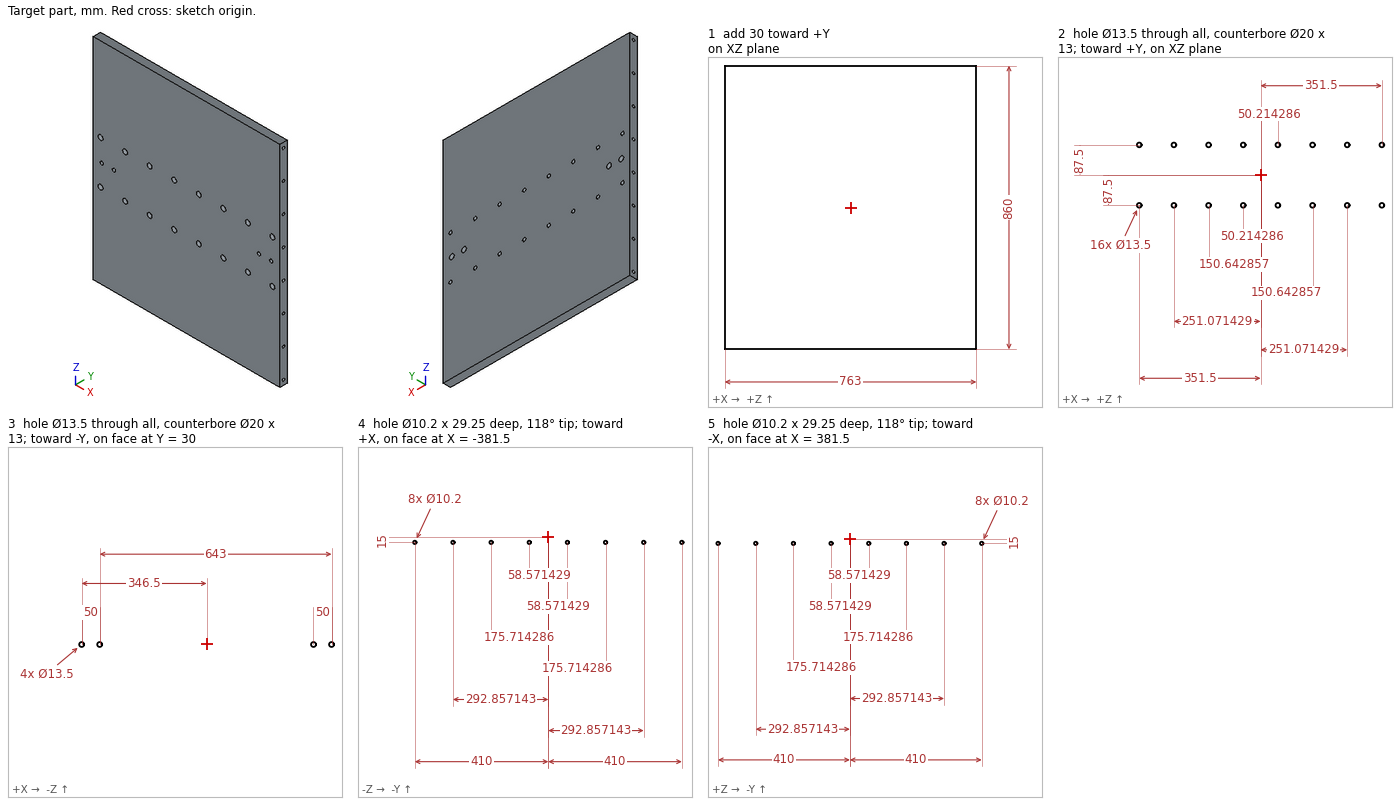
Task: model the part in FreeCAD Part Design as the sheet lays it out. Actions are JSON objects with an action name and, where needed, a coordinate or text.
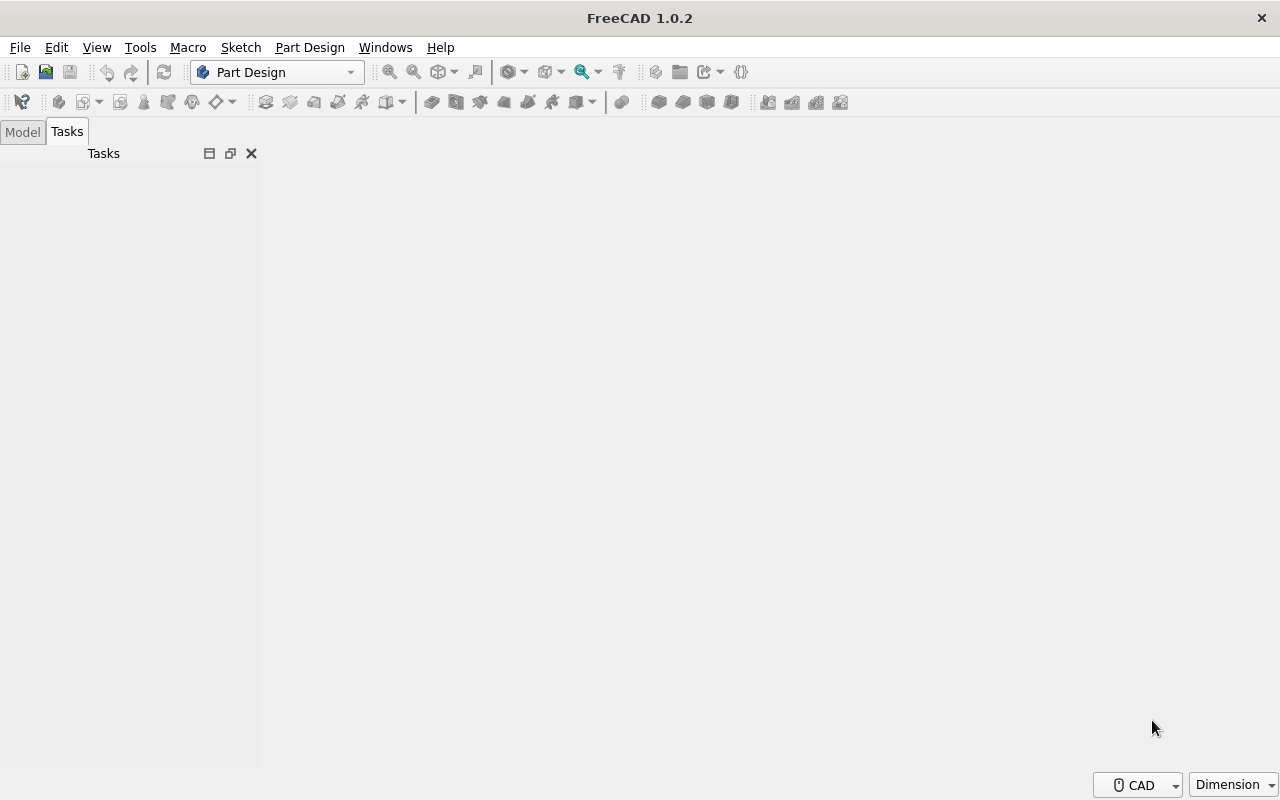
{"action": "left_click", "coordinate": [22, 72]}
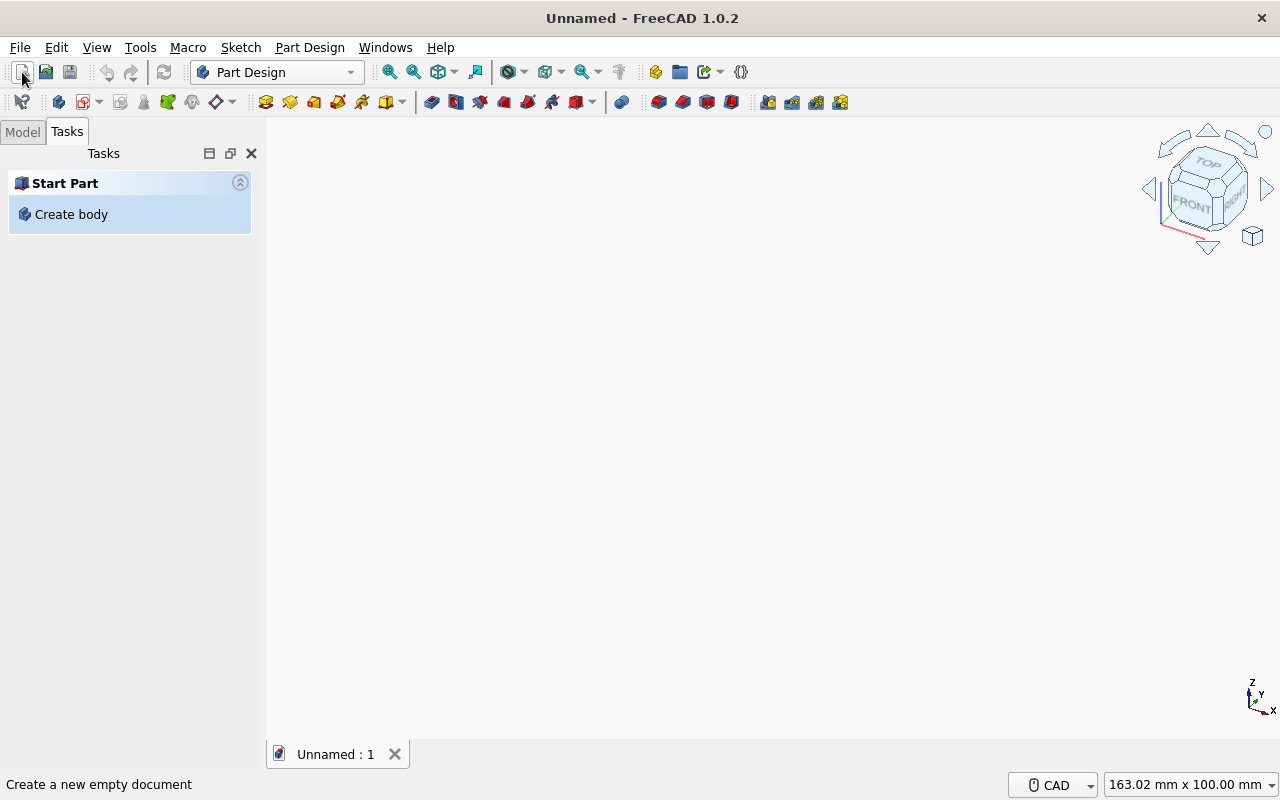
{"action": "left_click", "coordinate": [84, 102]}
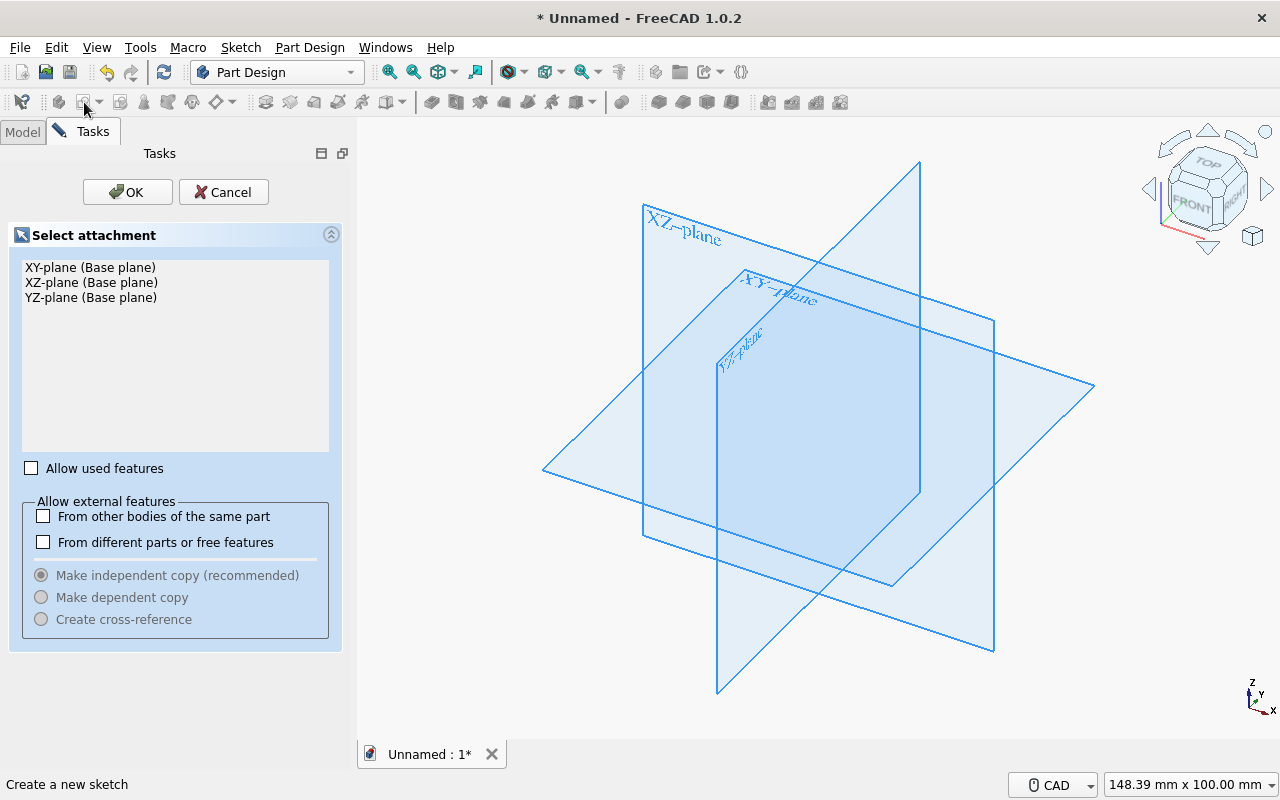
{"action": "left_click", "coordinate": [82, 282]}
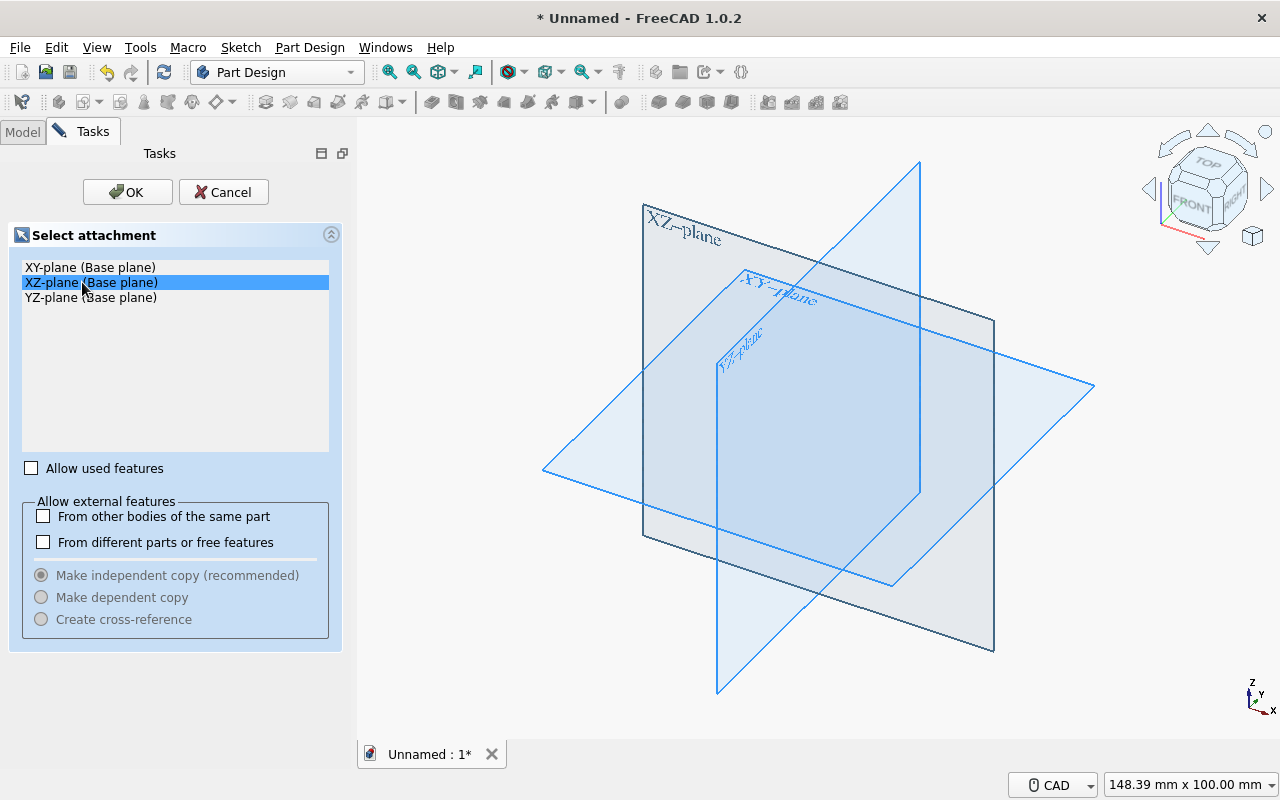
{"action": "left_click", "coordinate": [128, 192]}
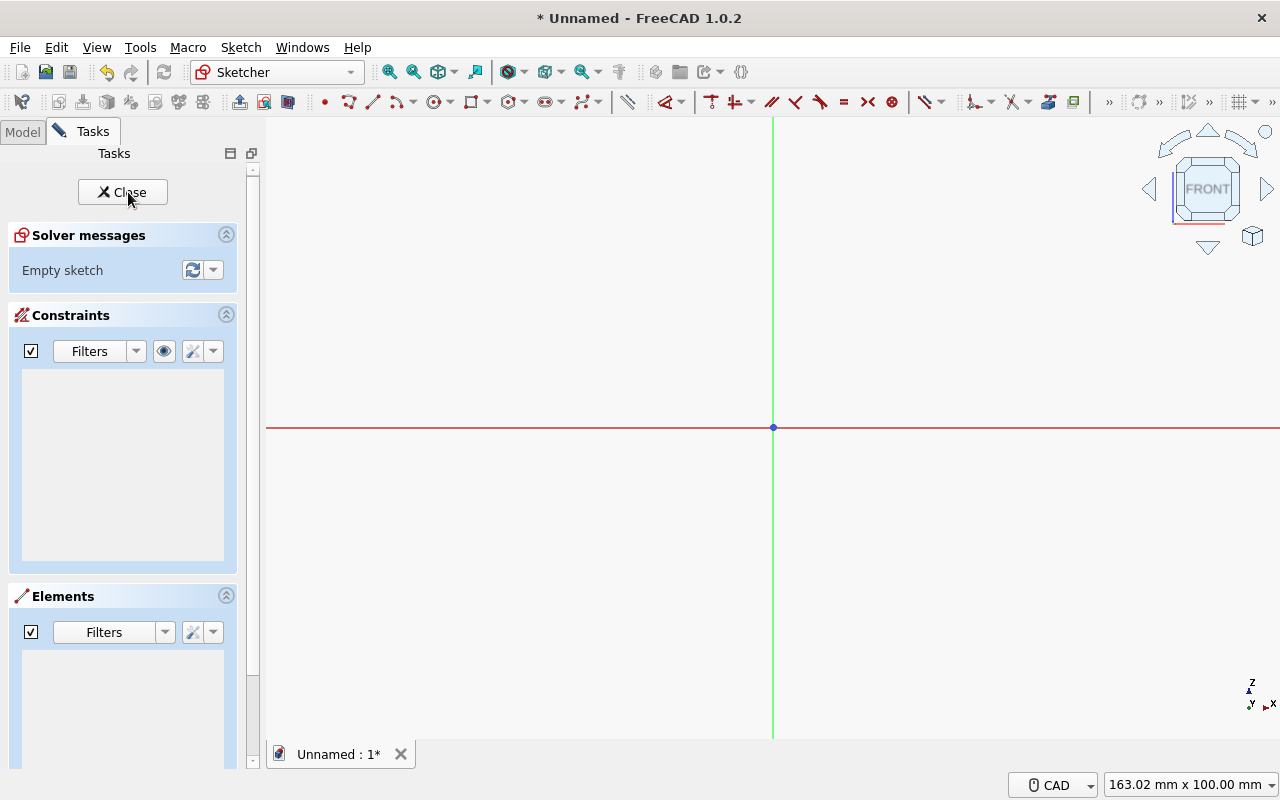
{"action": "scroll", "coordinate": [699, 428], "scroll_direction": "down", "scroll_amount": 13}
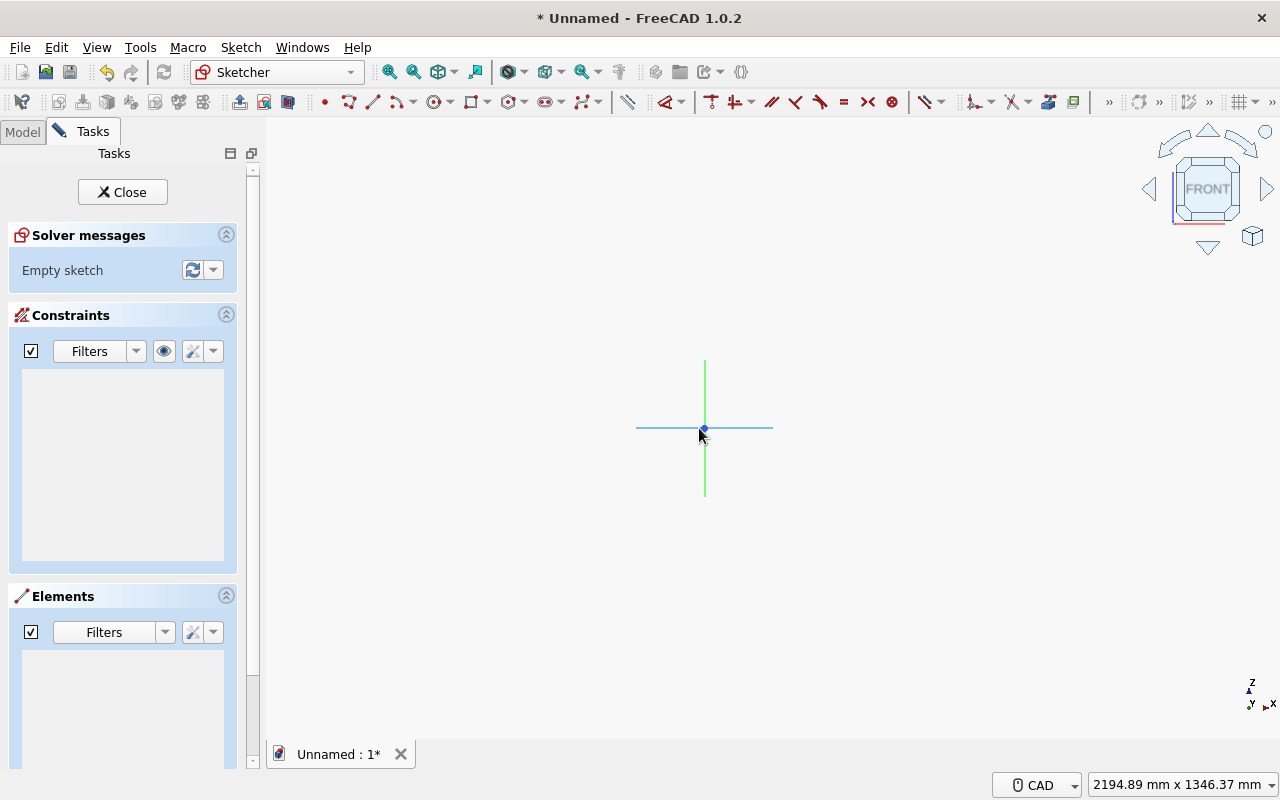
{"action": "left_click", "coordinate": [490, 102]}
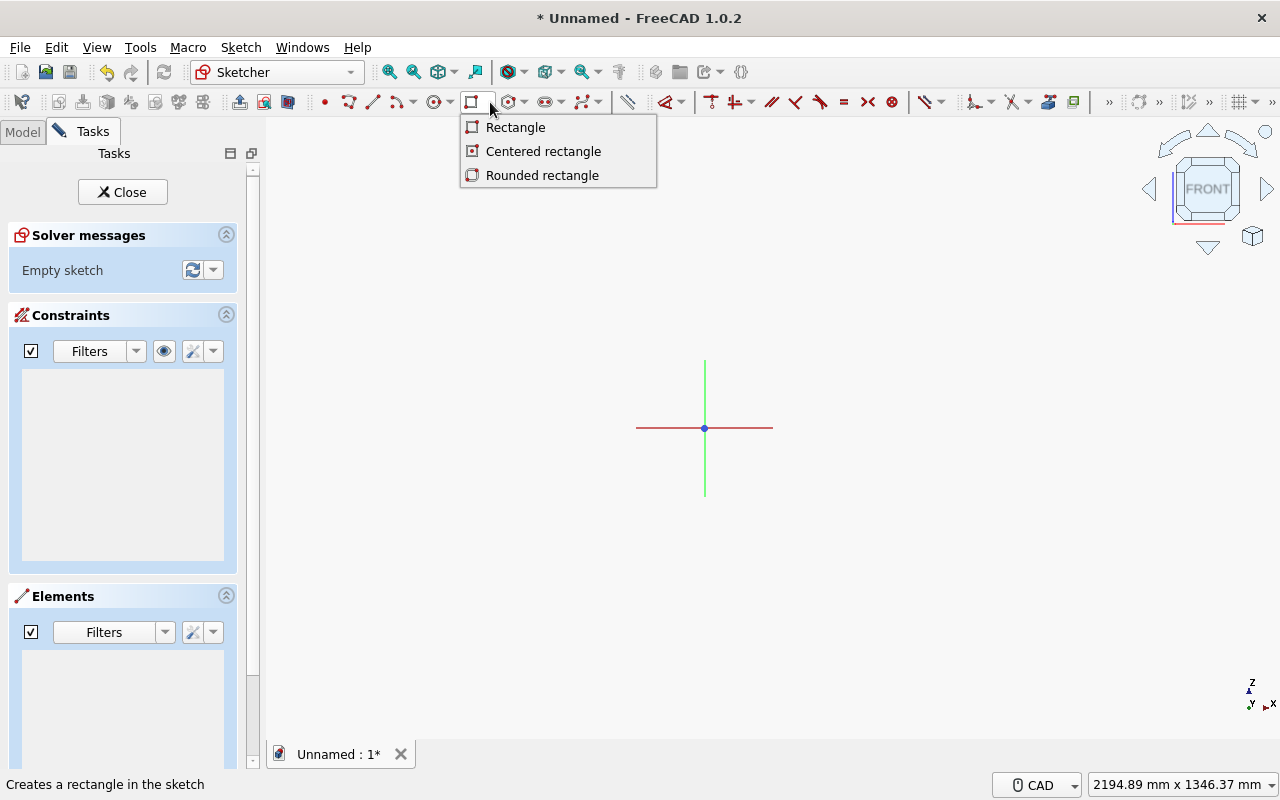
{"action": "left_click", "coordinate": [558, 151]}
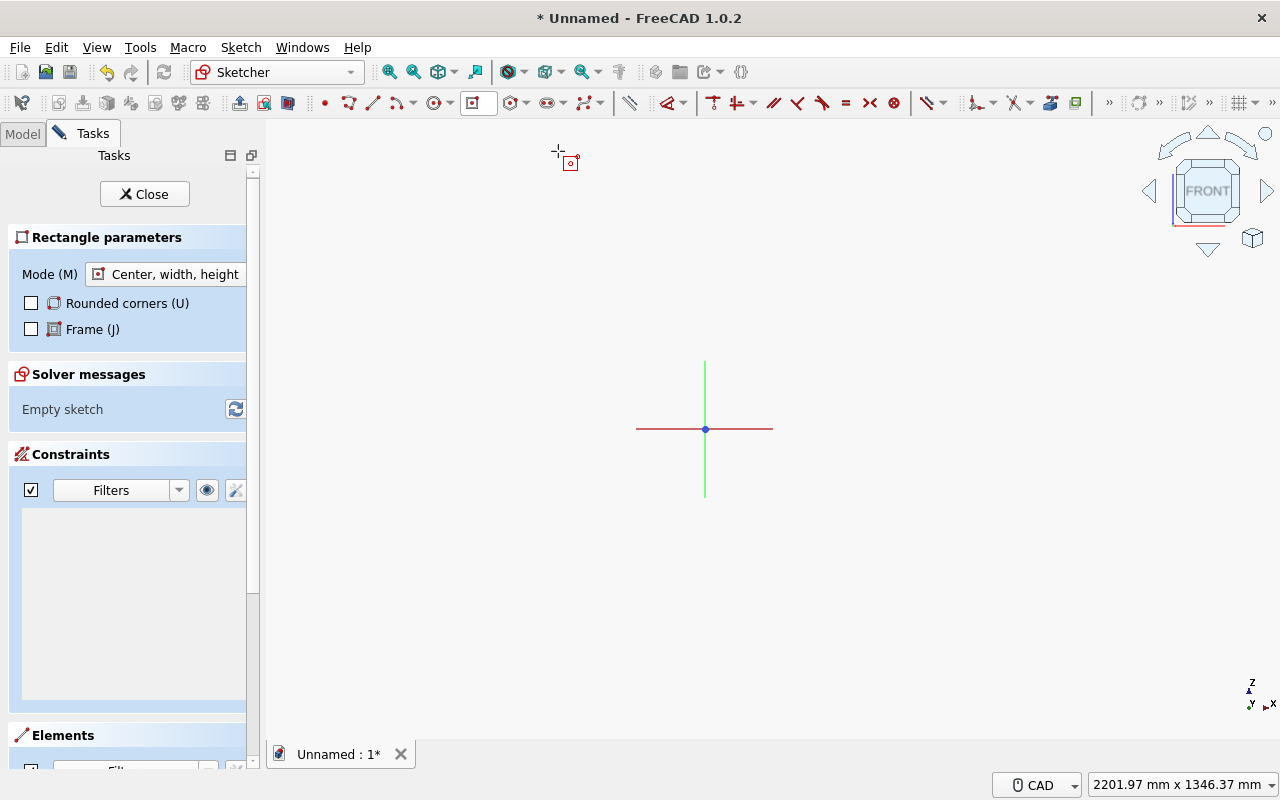
{"action": "left_click", "coordinate": [705, 429]}
{"action": "left_click", "coordinate": [881, 231]}
{"action": "key", "text": "Escape"}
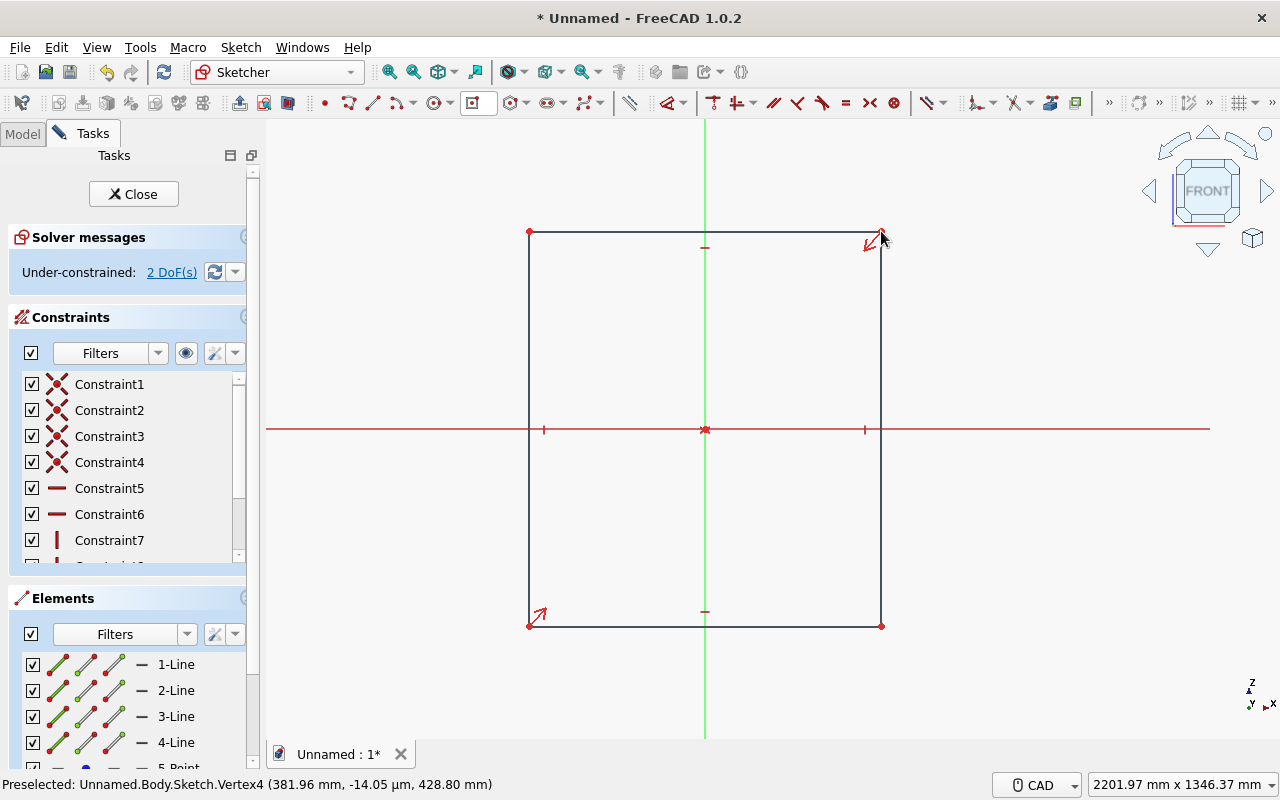
{"action": "left_click", "coordinate": [635, 627]}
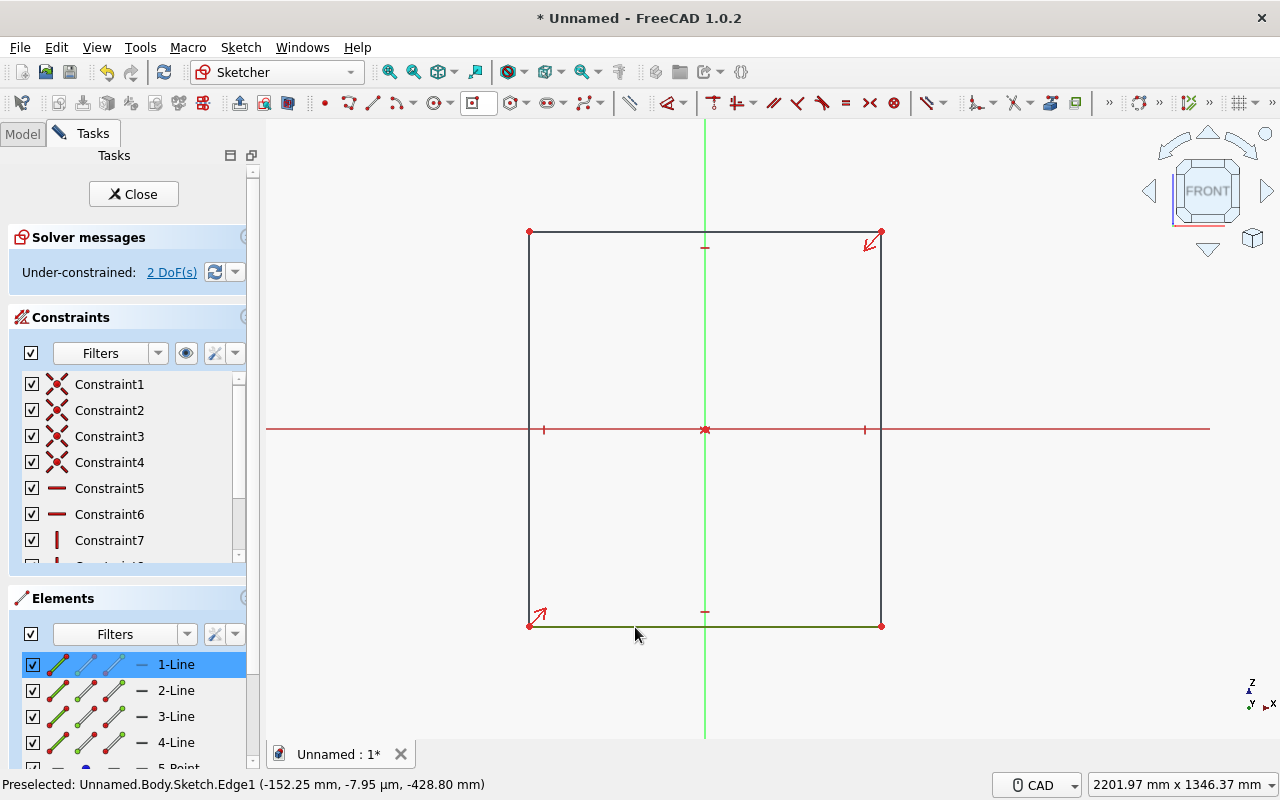
{"action": "left_click", "coordinate": [686, 104]}